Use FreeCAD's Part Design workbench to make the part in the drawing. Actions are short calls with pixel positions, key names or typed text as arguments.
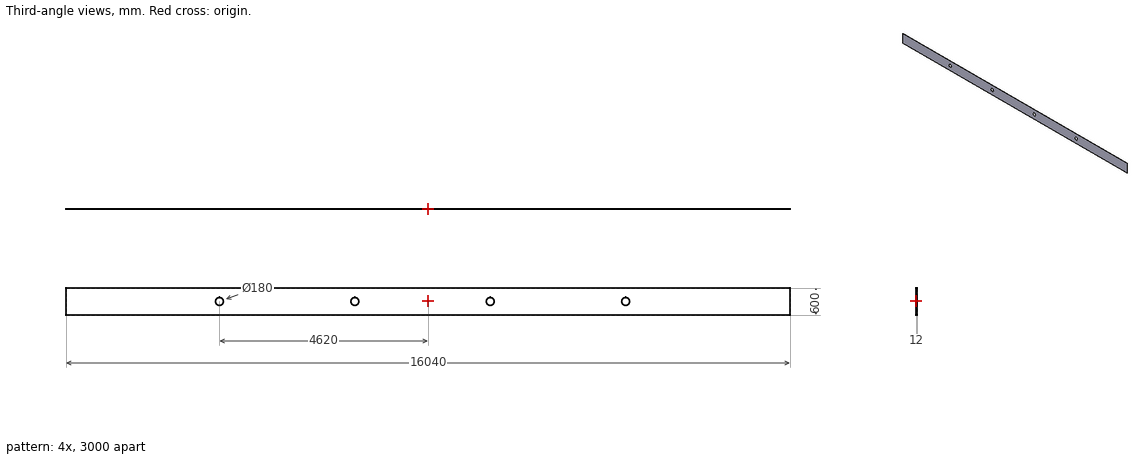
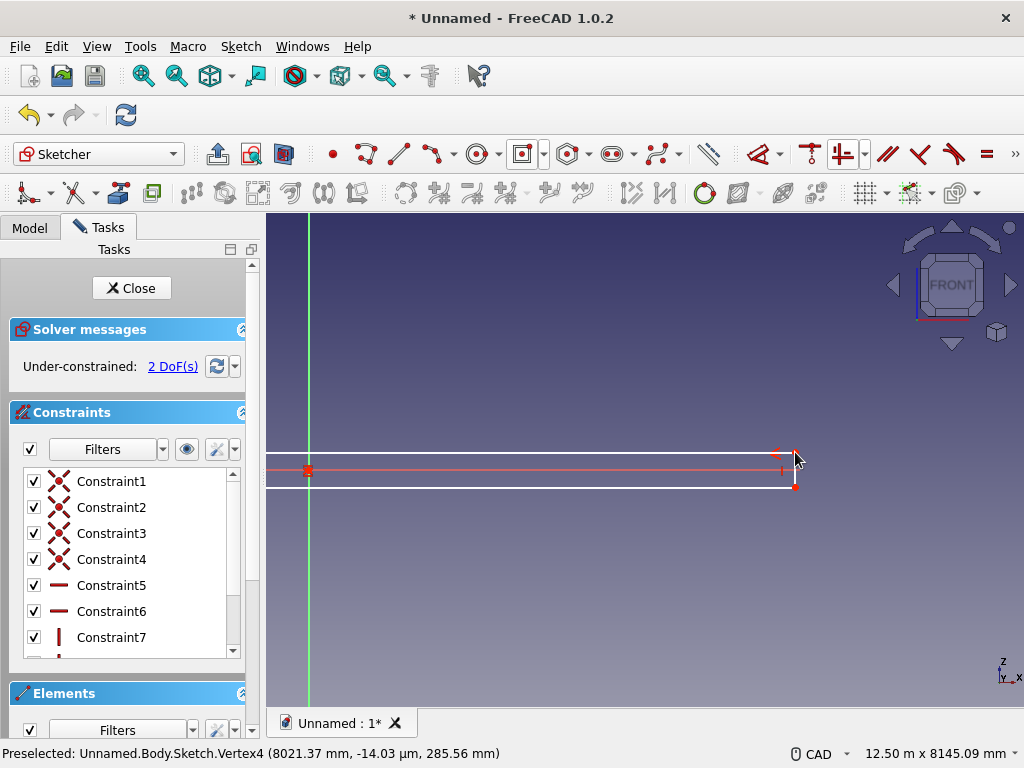
click(758, 154)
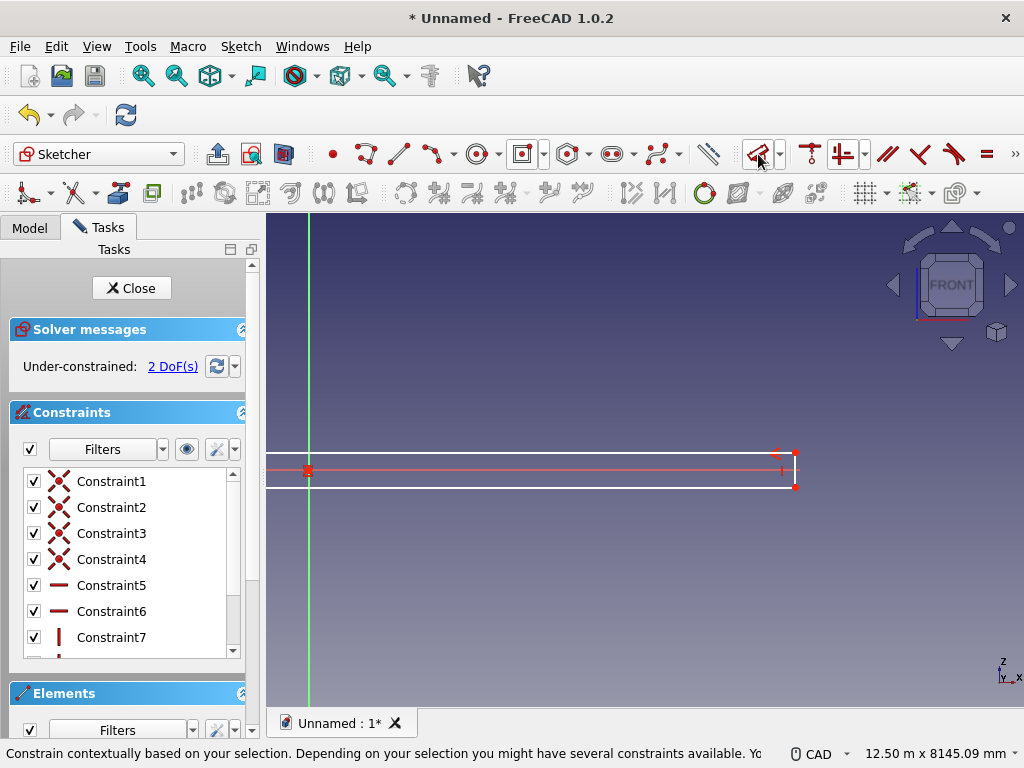
click(795, 474)
click(829, 462)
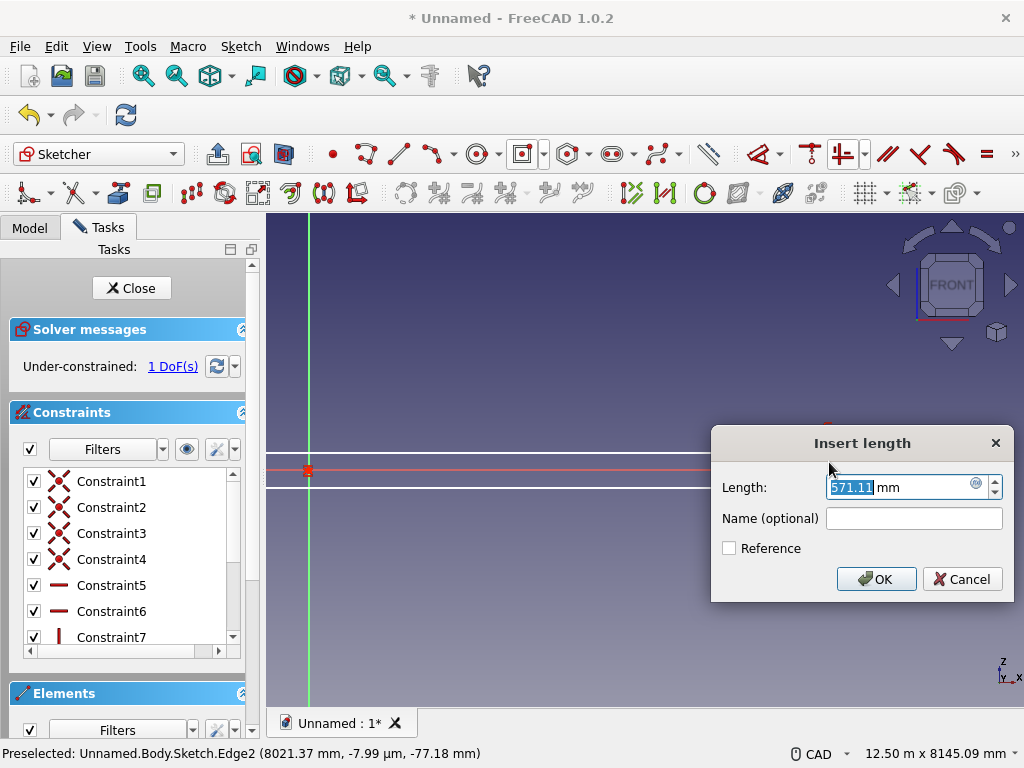
text(600)
key(Return)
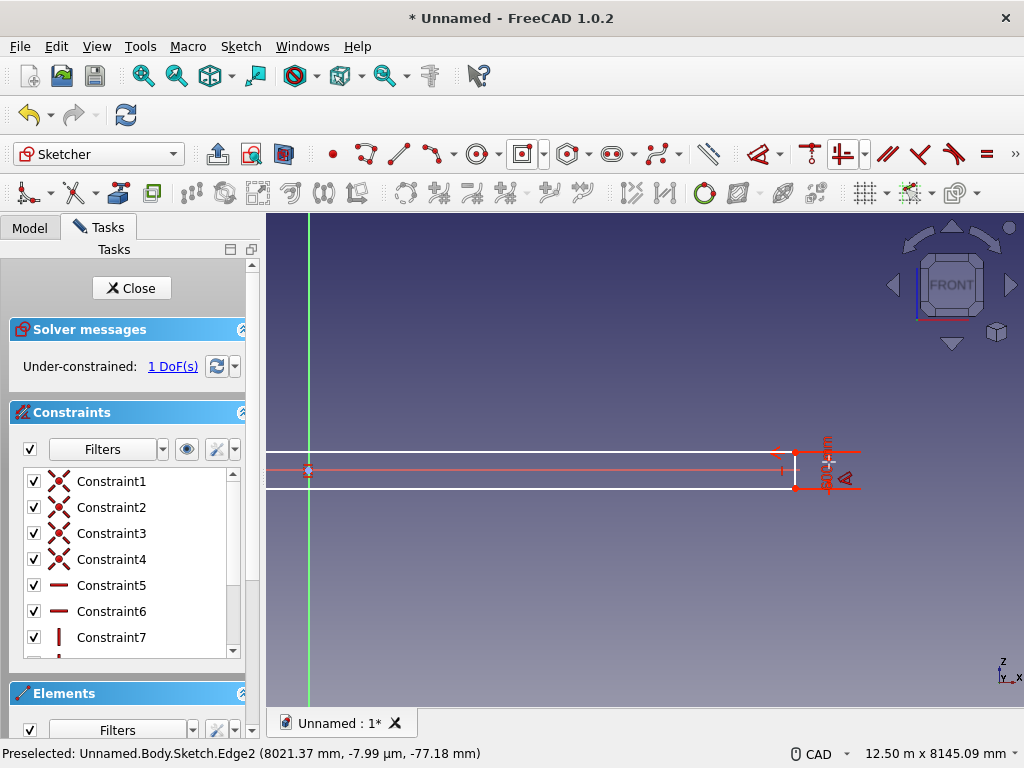
click(503, 489)
click(545, 523)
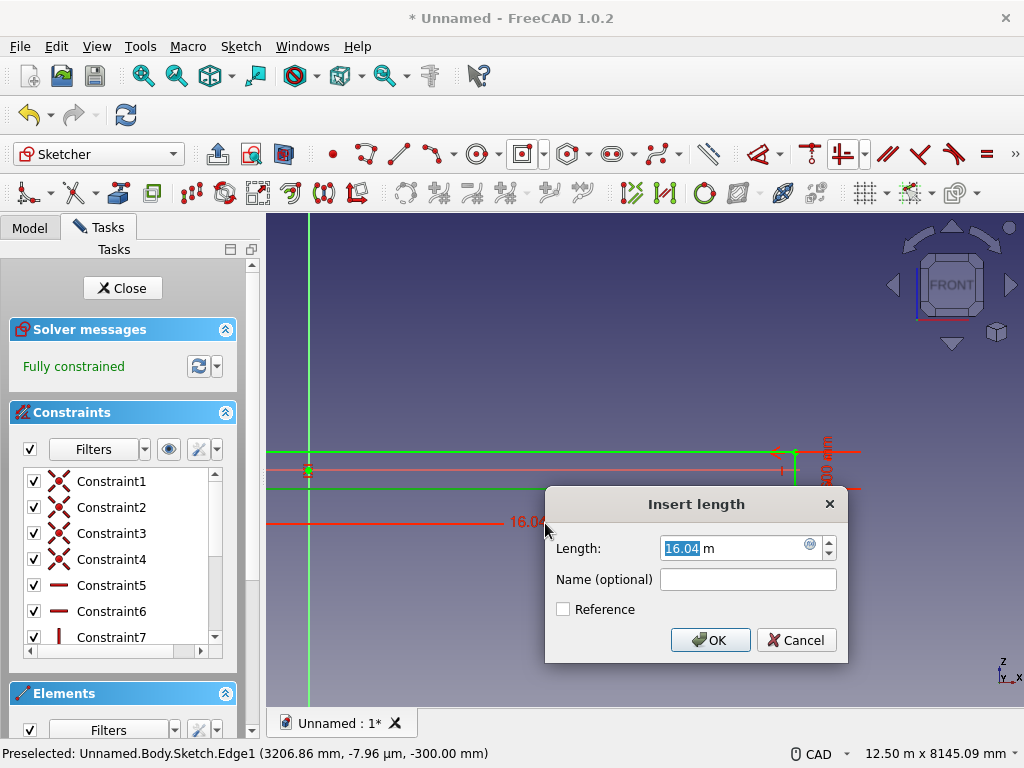
key(ctrl+a)
text(16040 mm)
key(Return)
key(Escape)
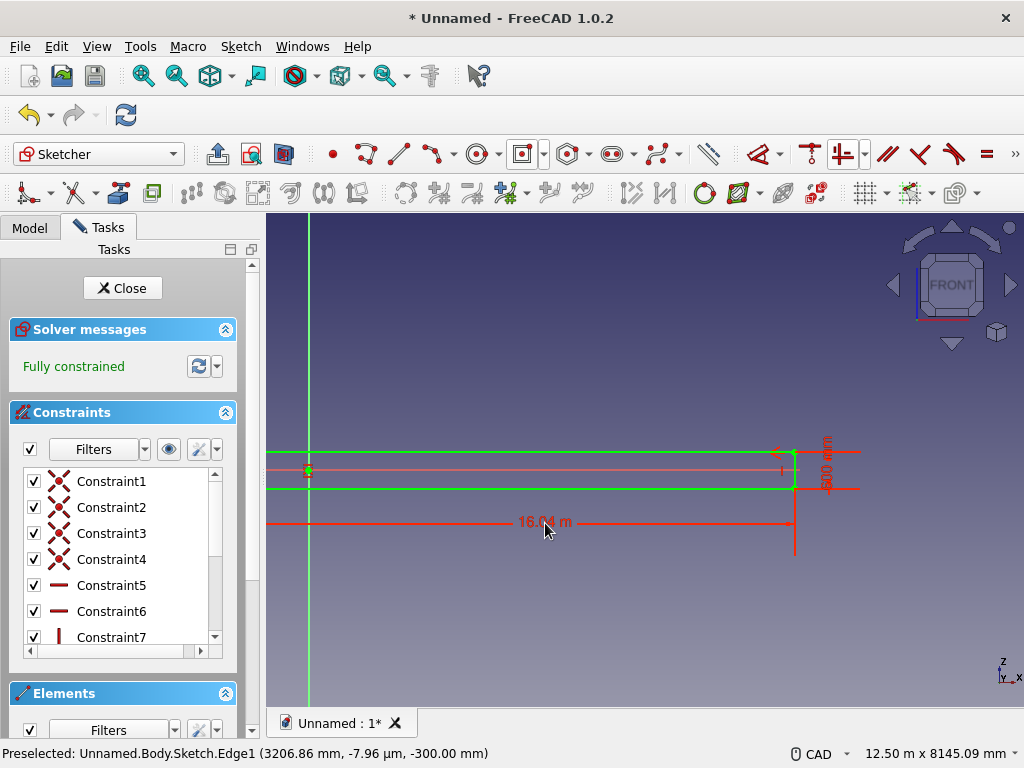
click(123, 288)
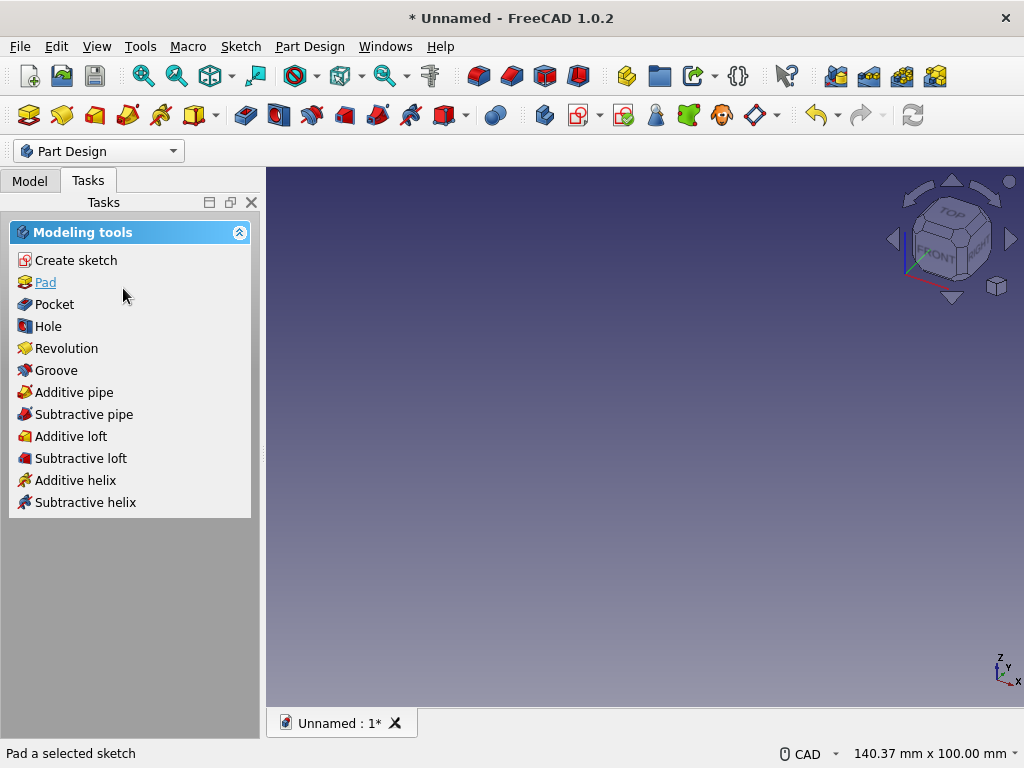
click(29, 116)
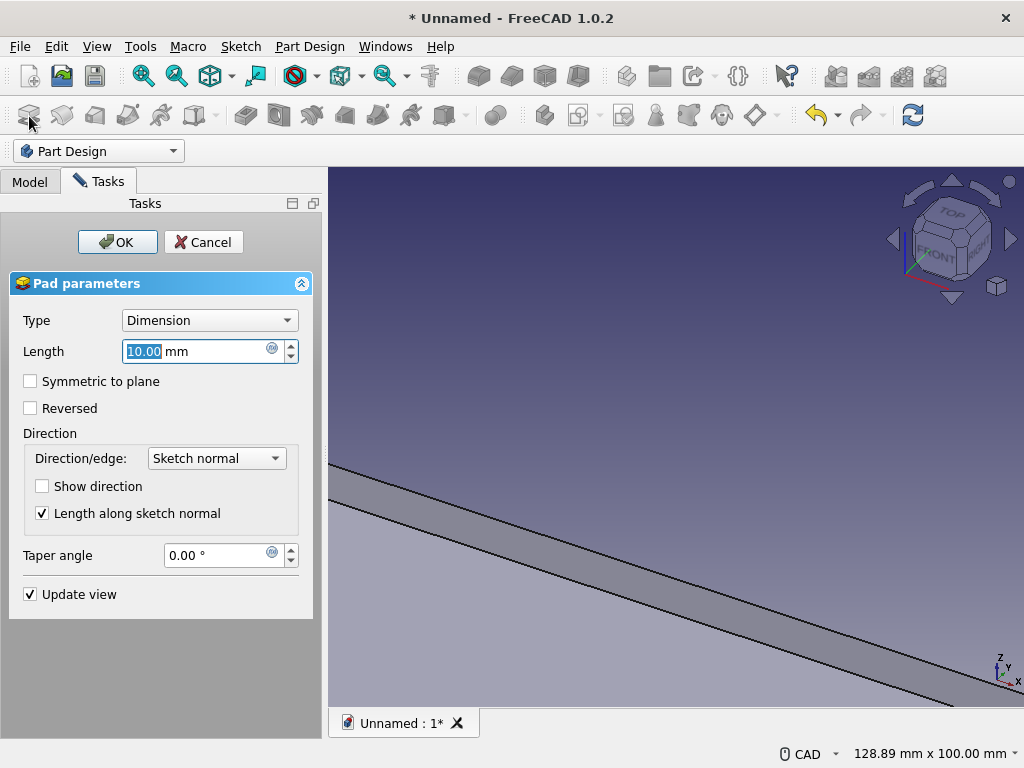
text(12)
key(Tab)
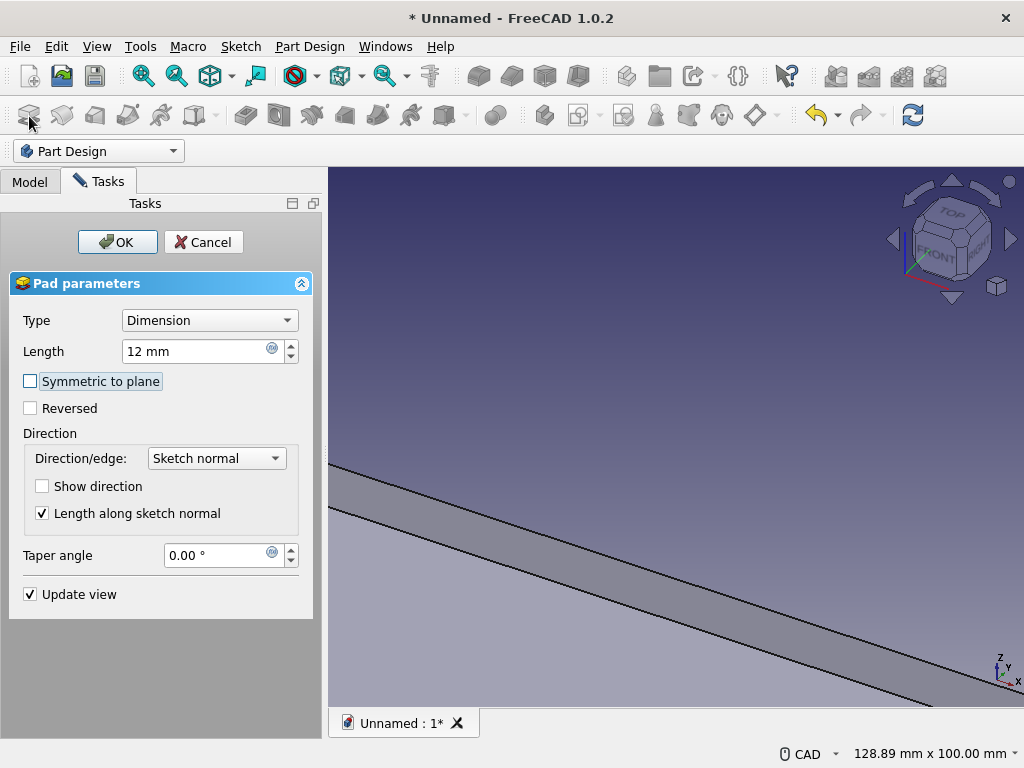
click(31, 408)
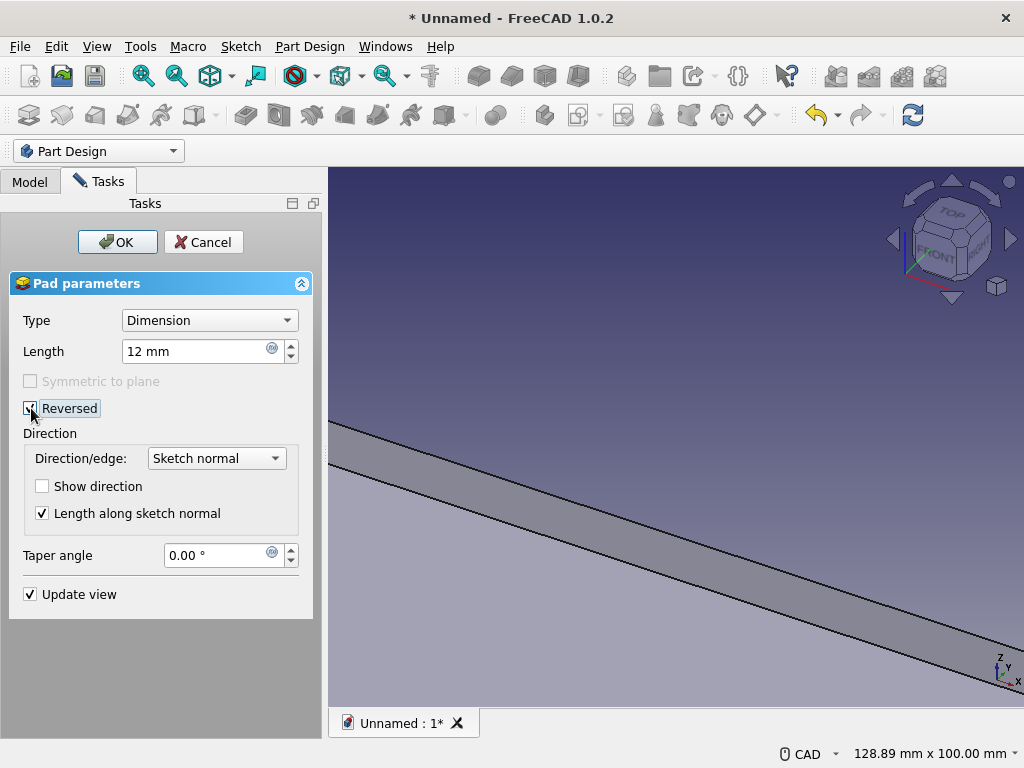
click(118, 242)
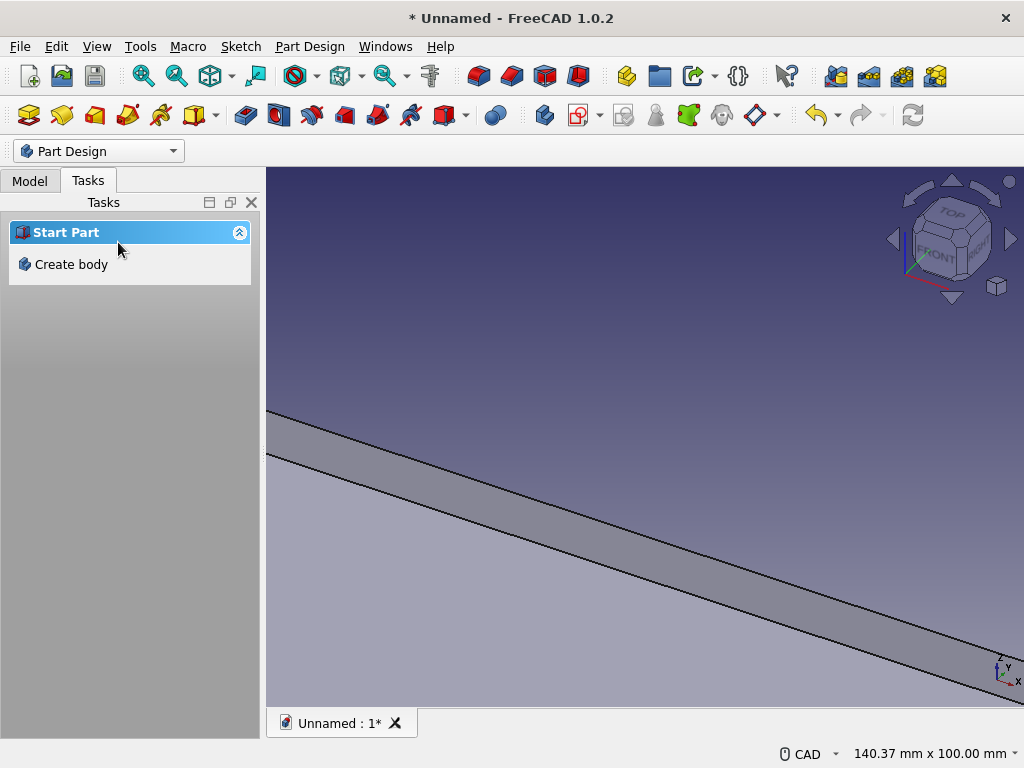
click(144, 76)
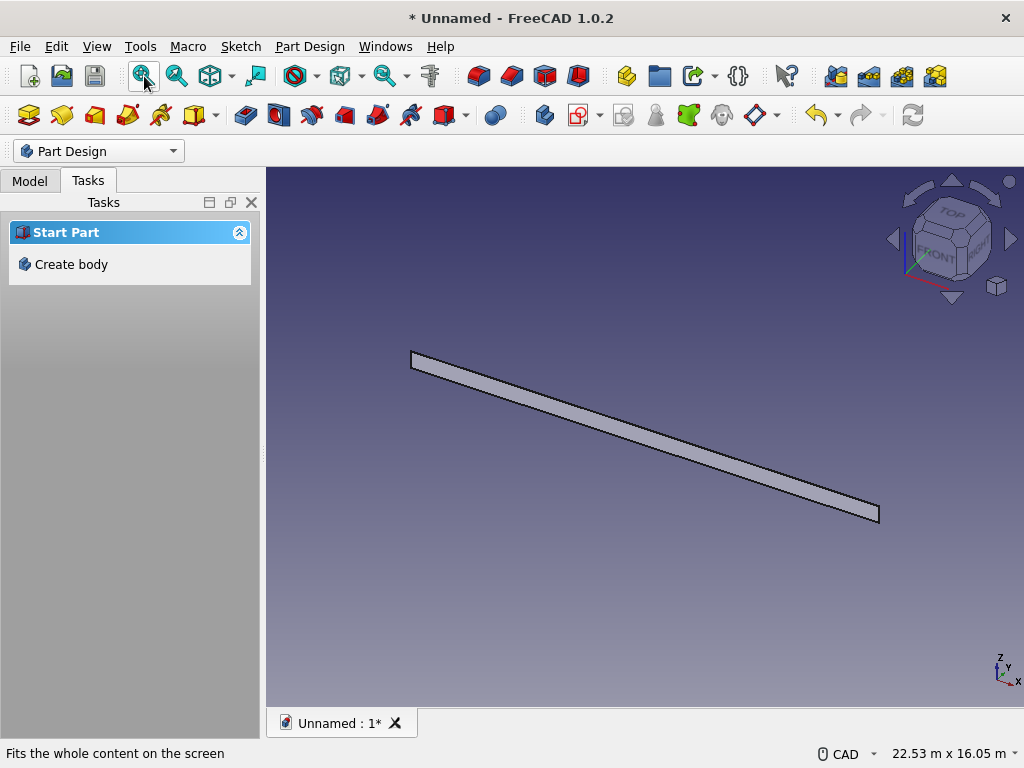
key(4)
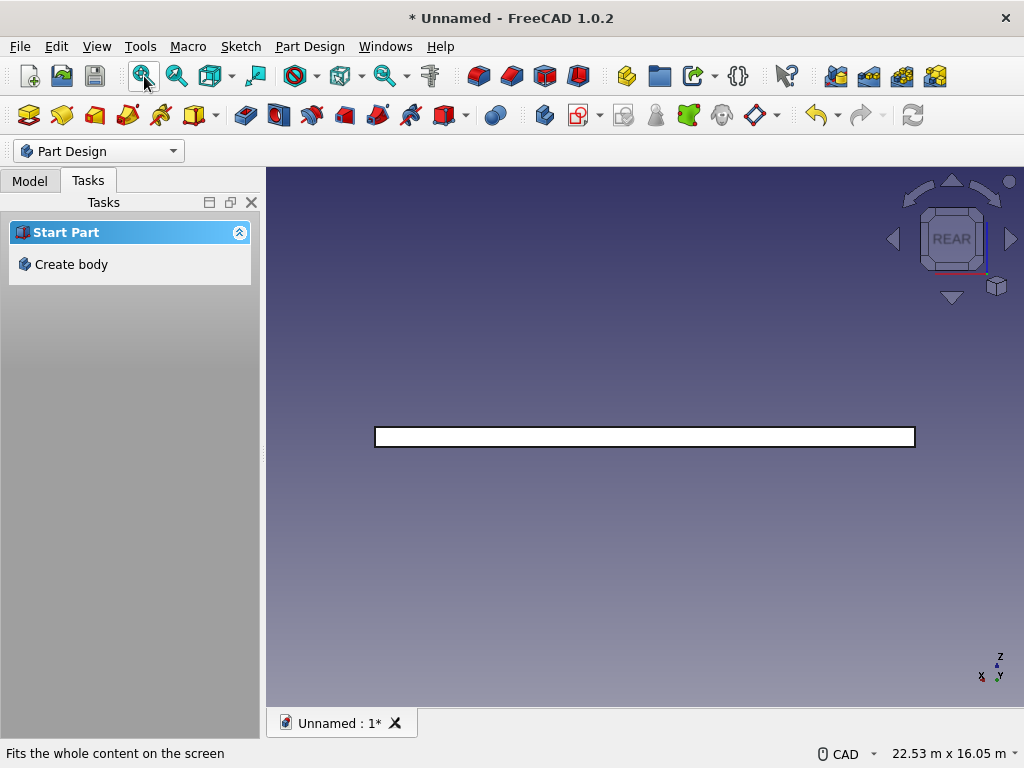
click(414, 436)